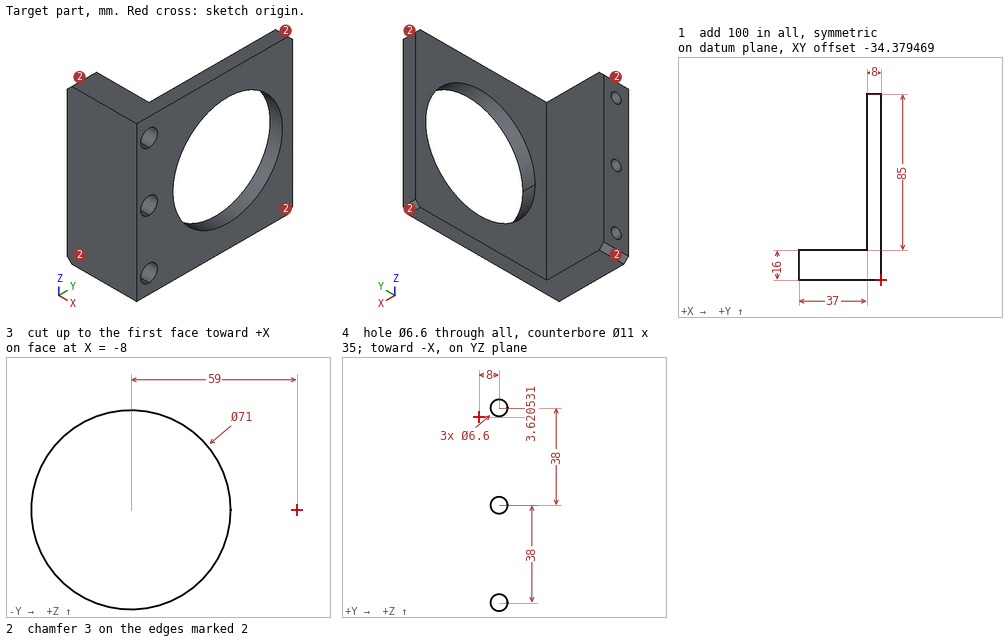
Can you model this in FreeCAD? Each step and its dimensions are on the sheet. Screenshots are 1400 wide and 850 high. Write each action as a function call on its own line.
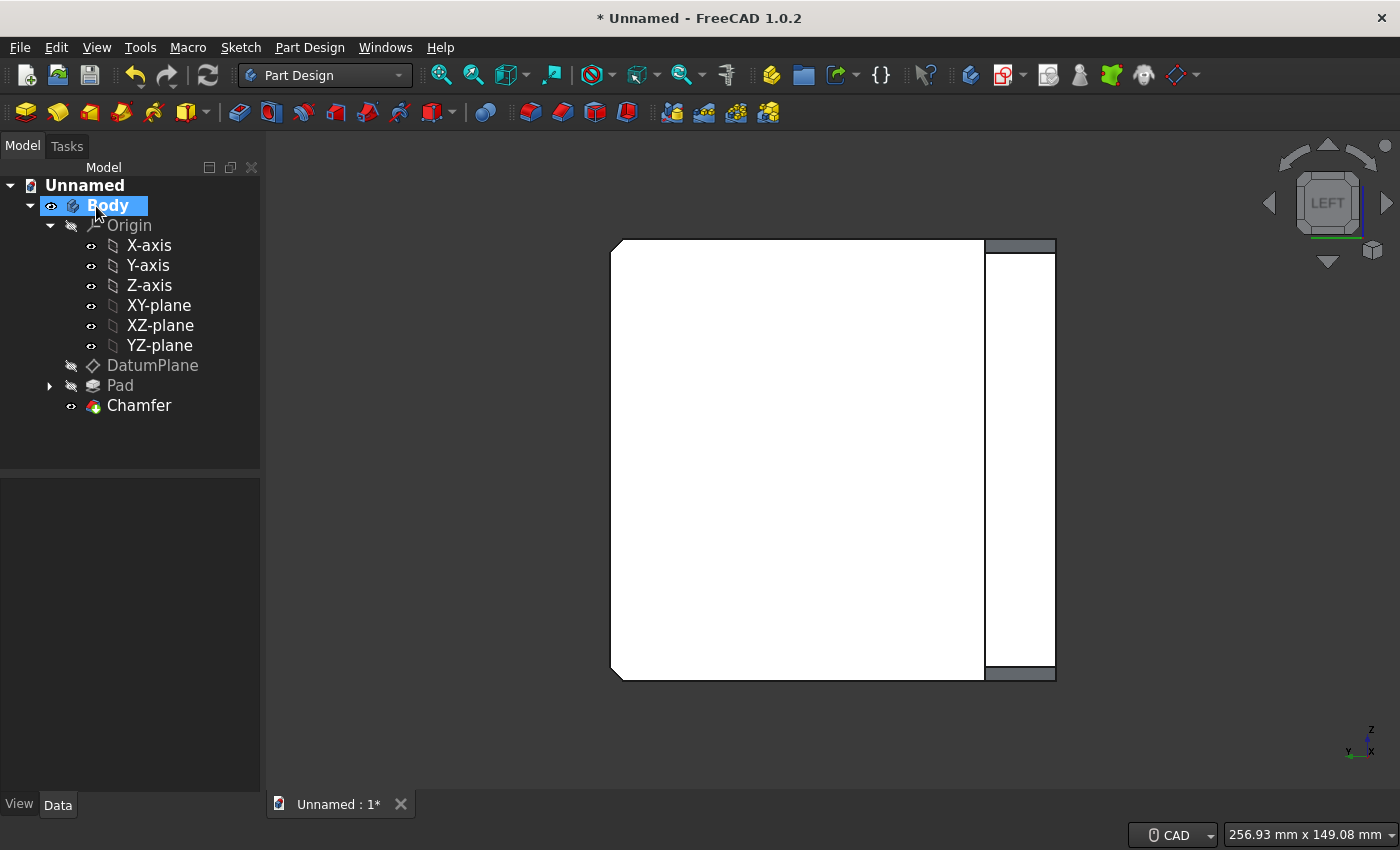
click(798, 459)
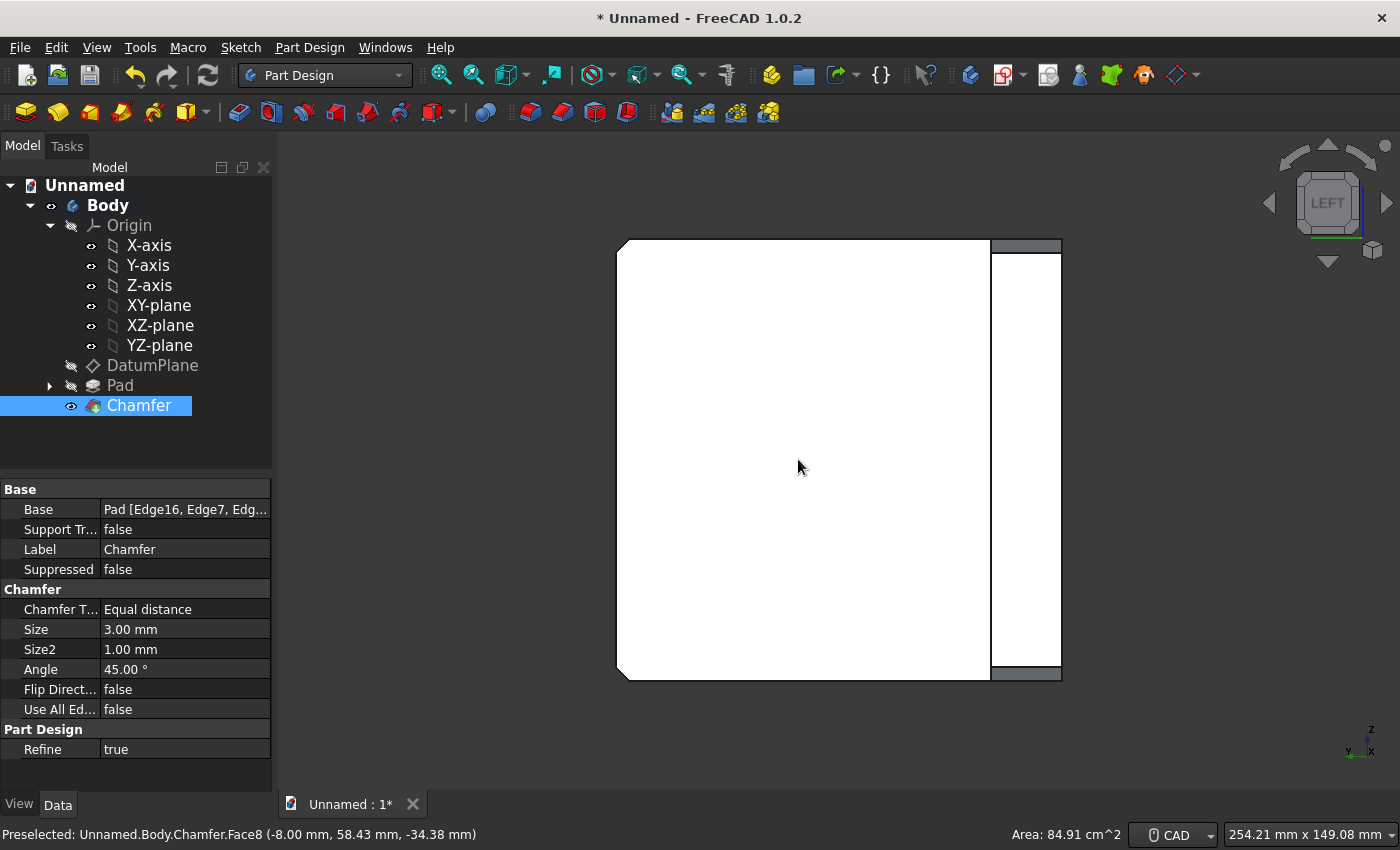
click(1004, 76)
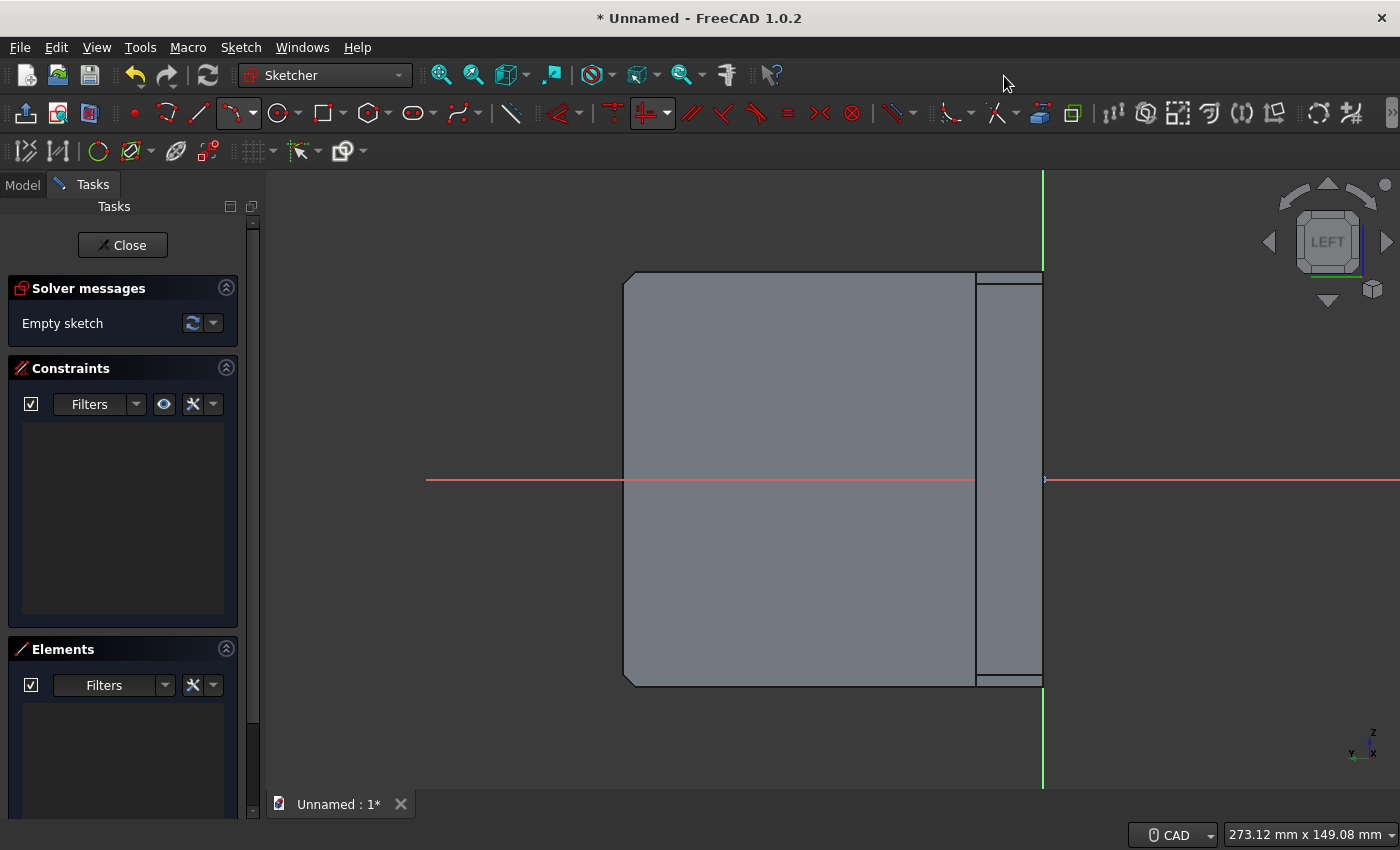
click(278, 114)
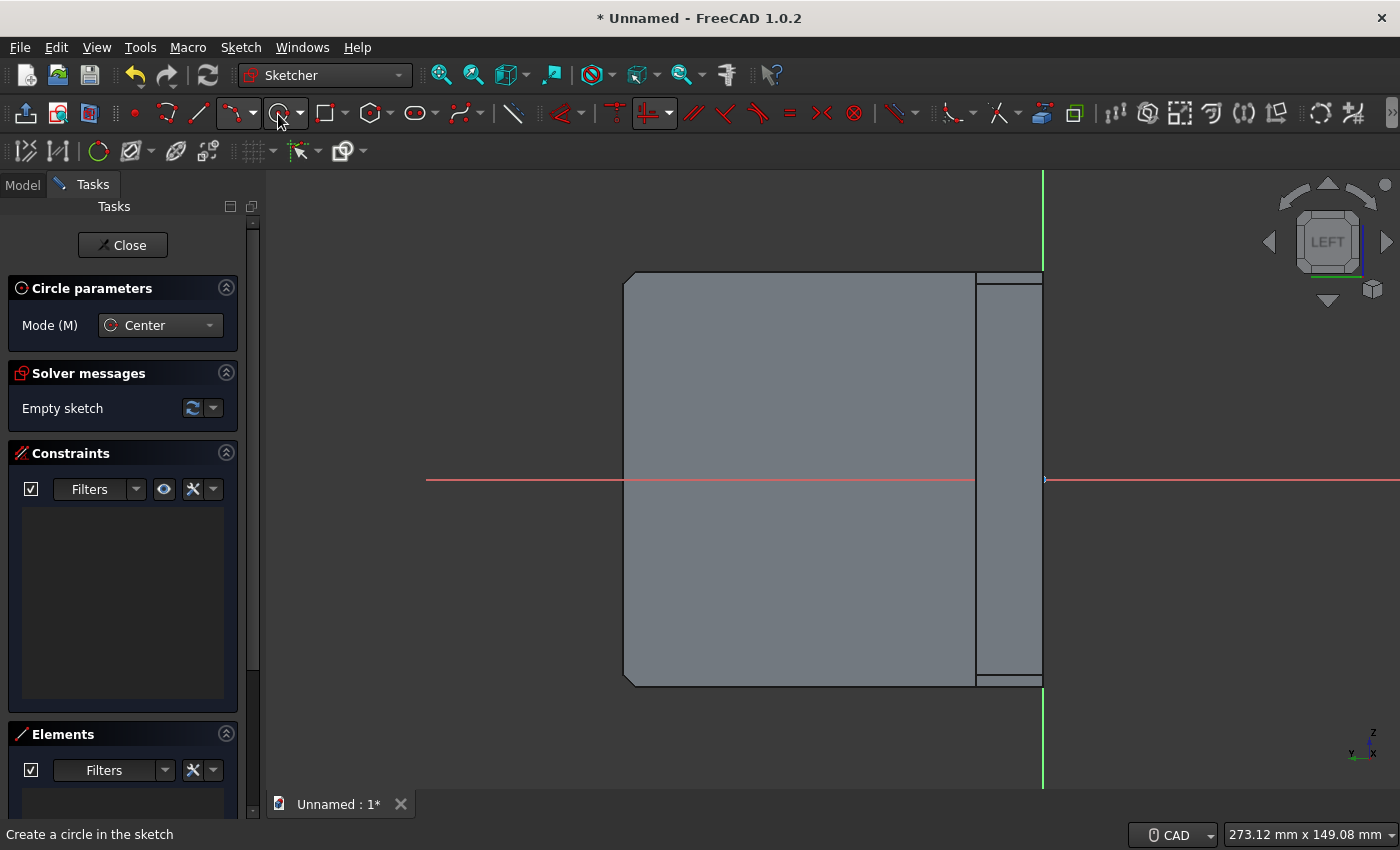
click(798, 479)
click(902, 375)
key(Escape)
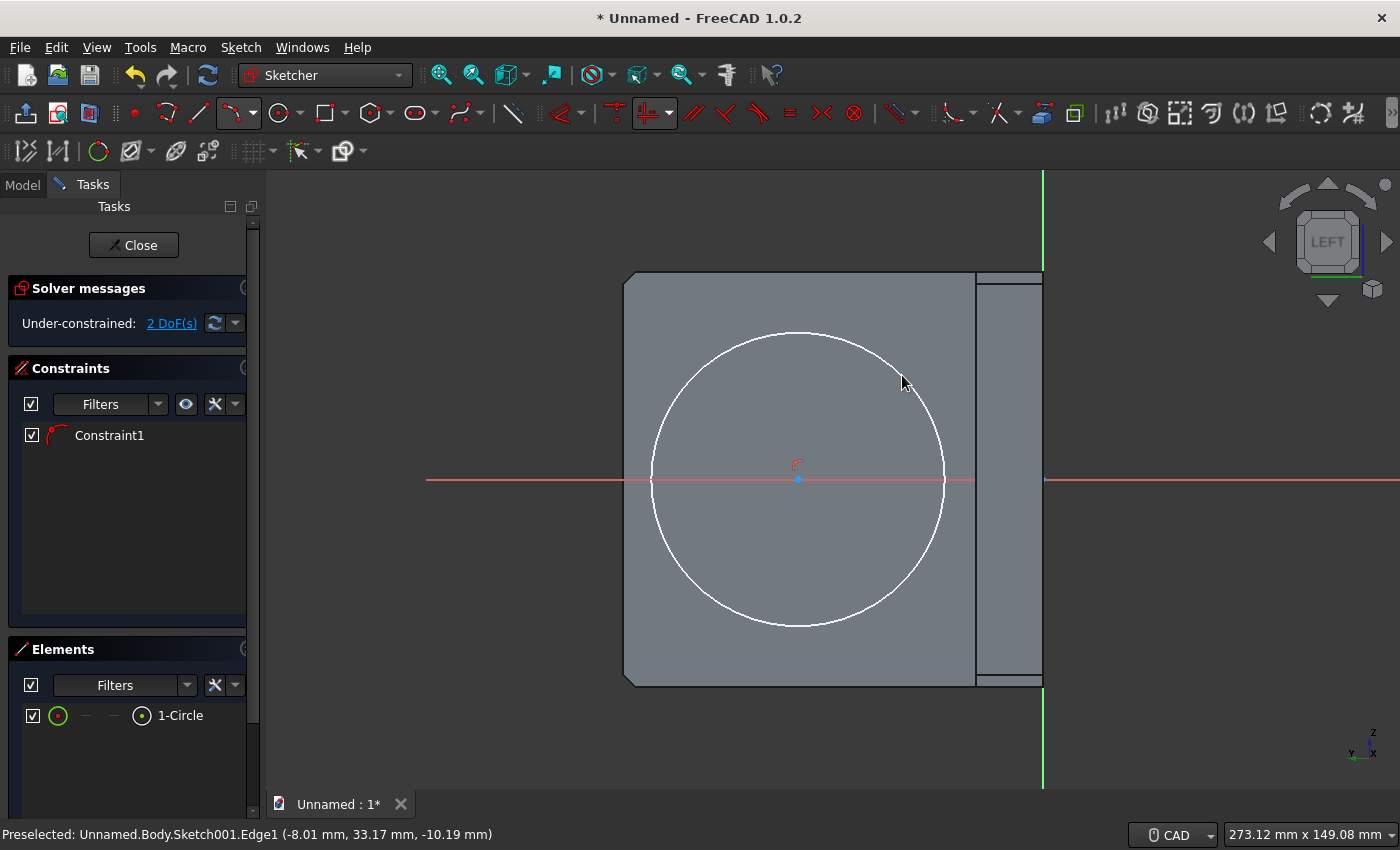
click(560, 114)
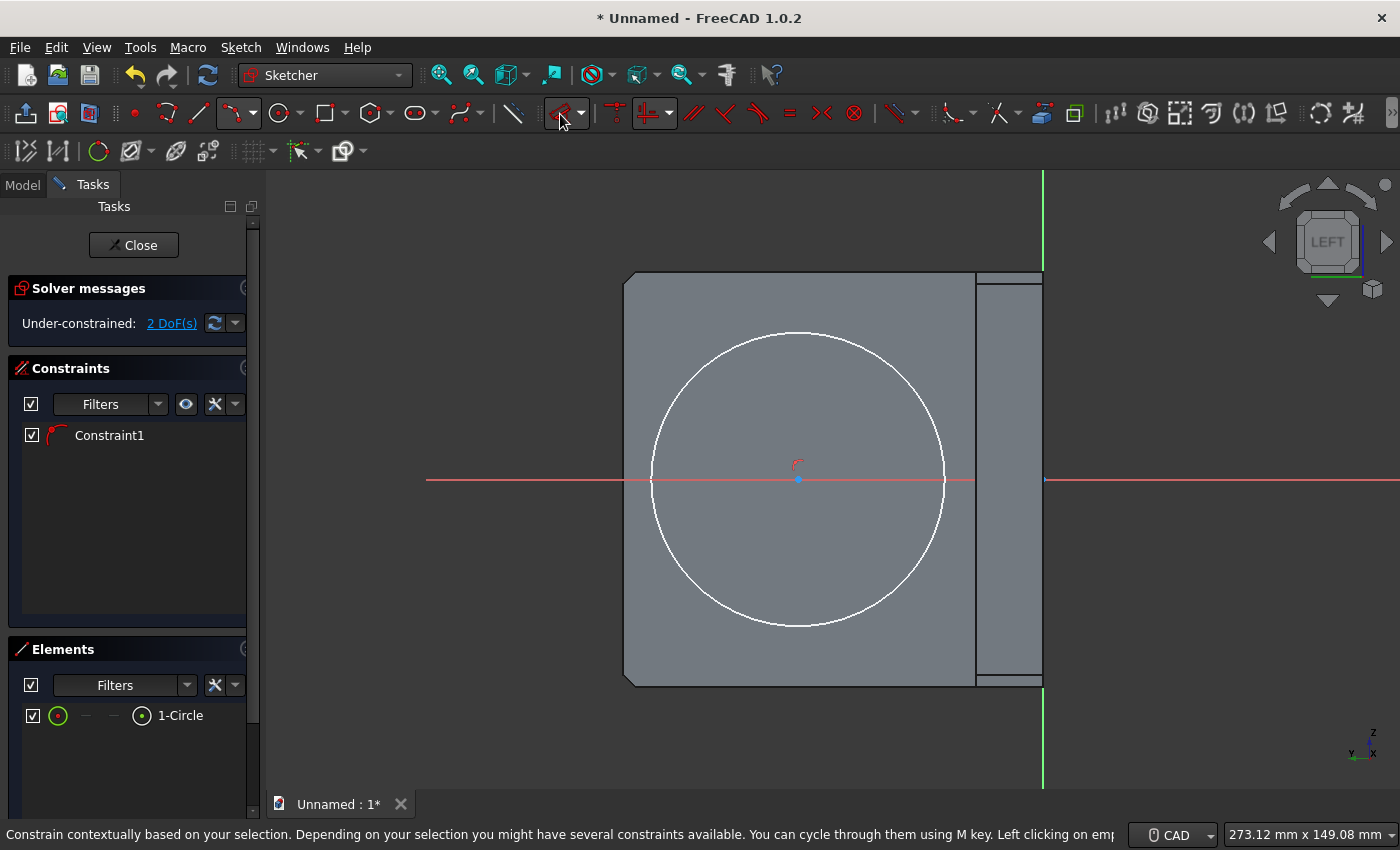
click(901, 375)
click(923, 352)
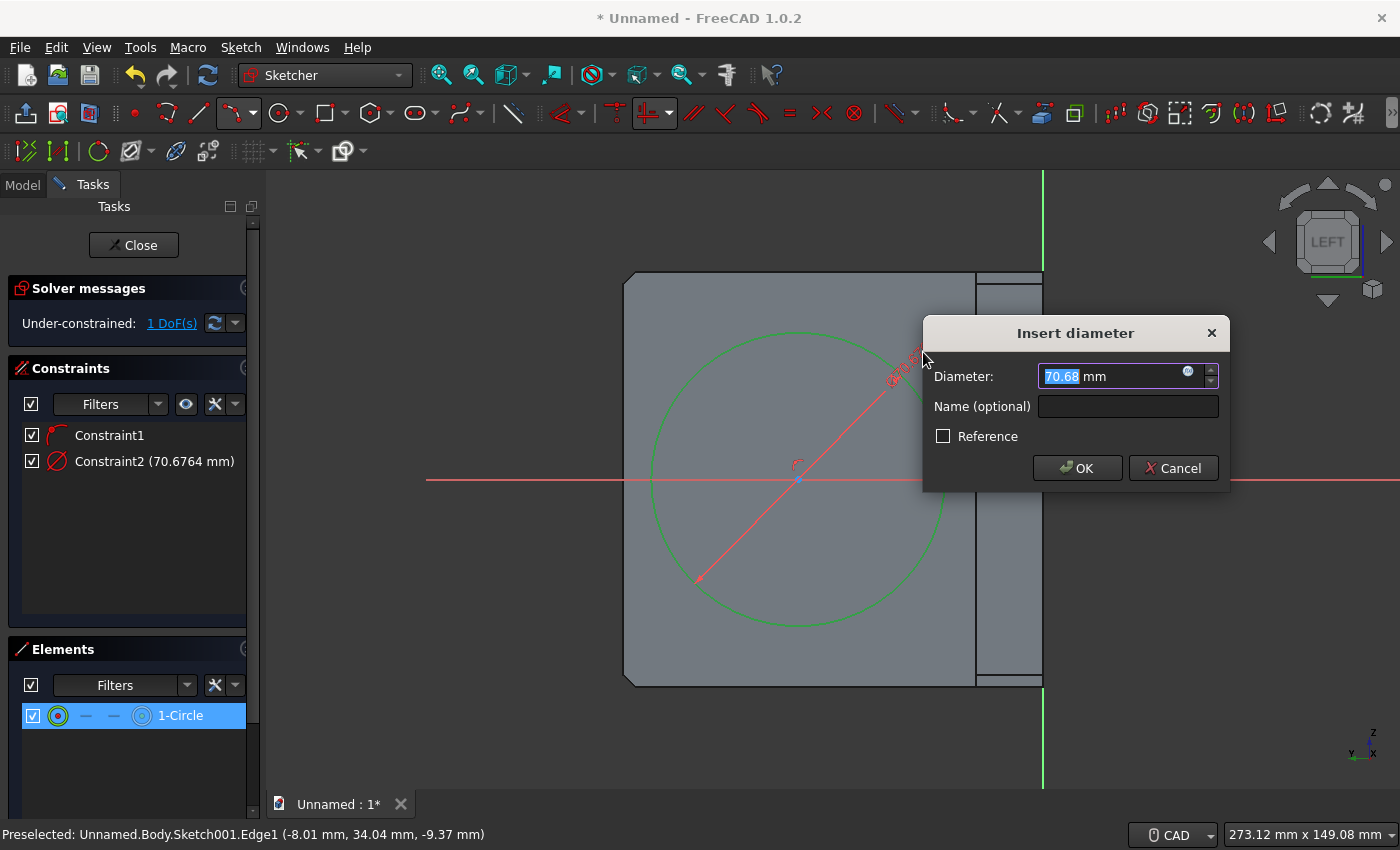
text(71)
key(Return)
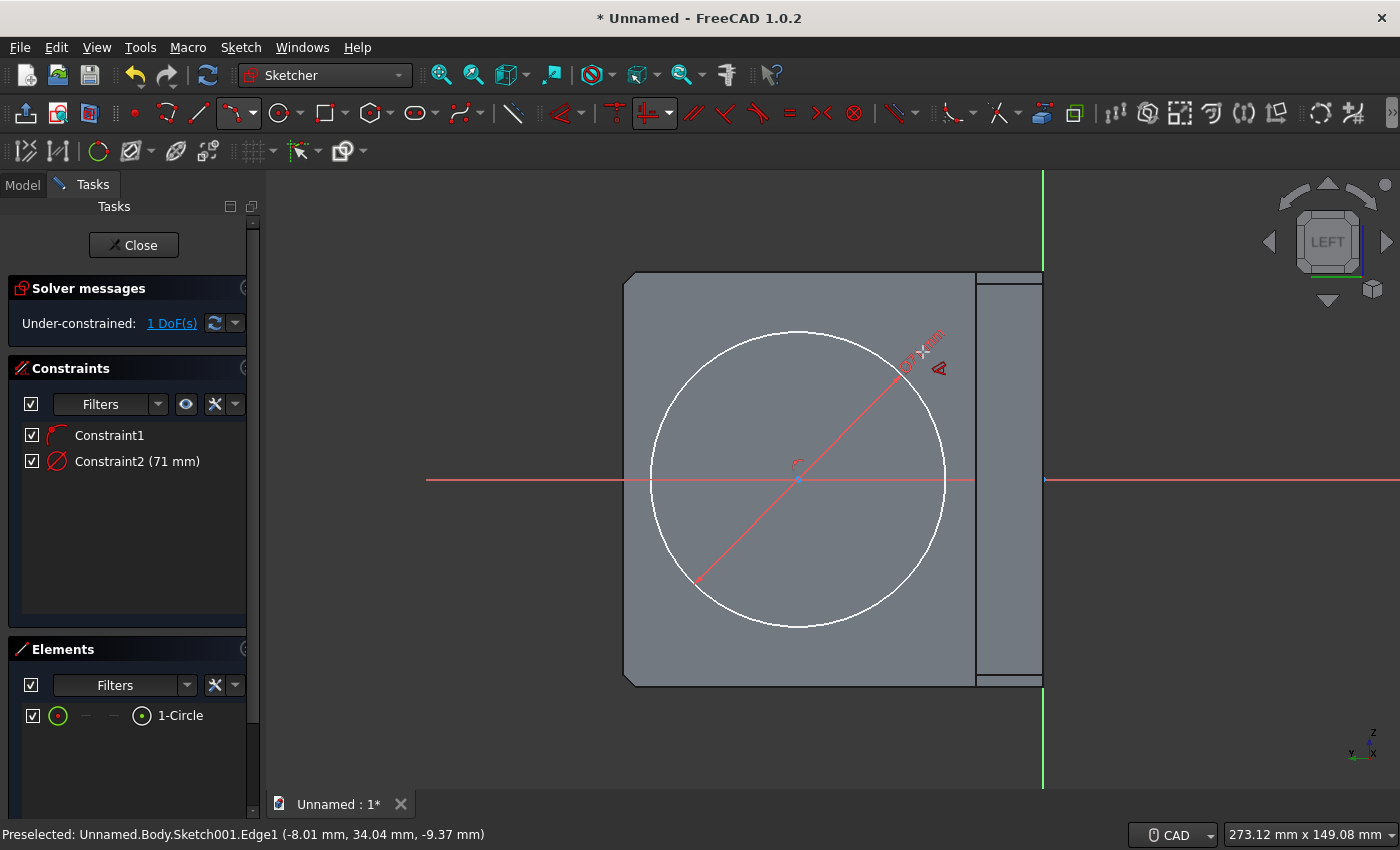
click(798, 479)
click(920, 513)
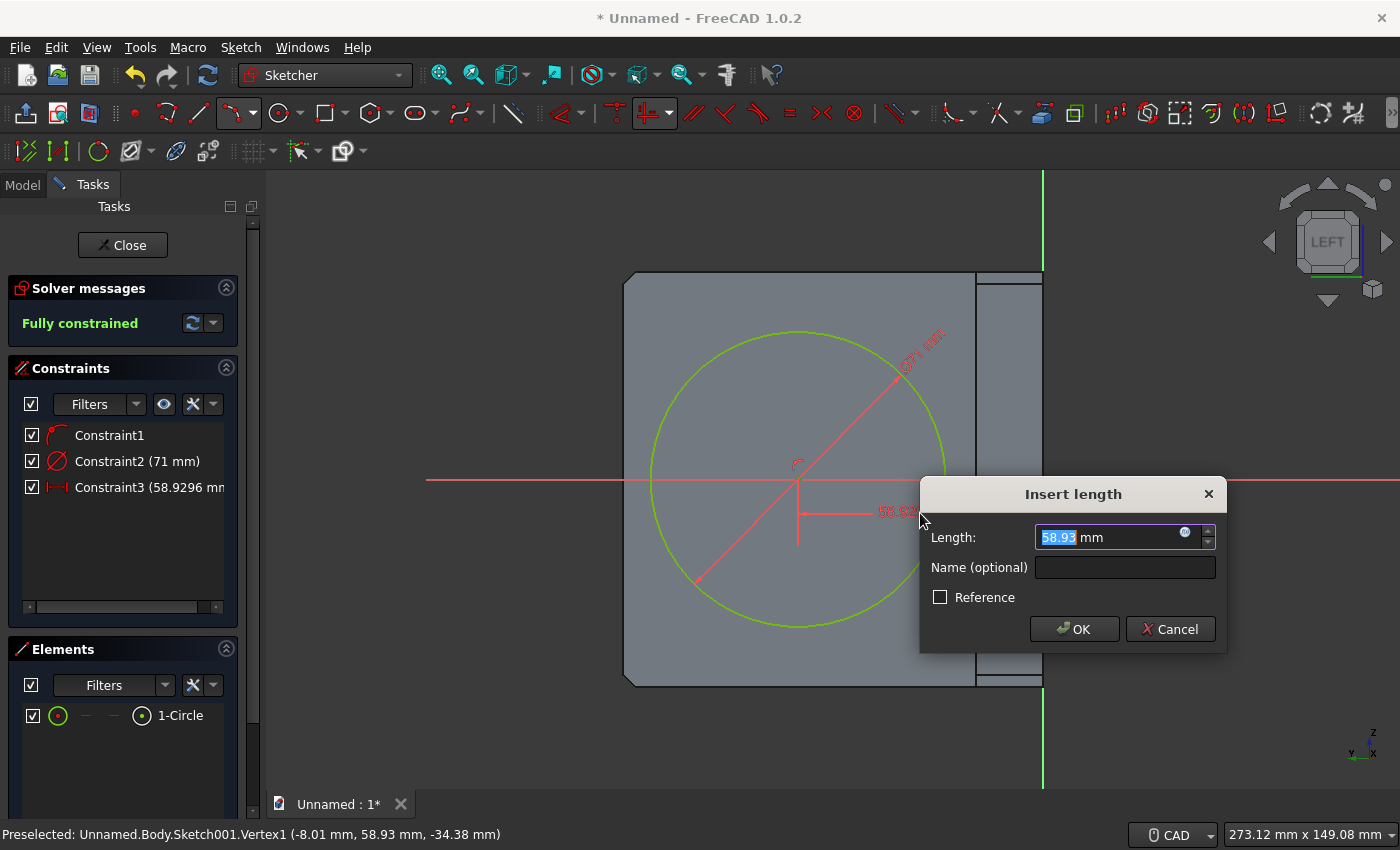
text(59)
key(Return)
key(Escape)